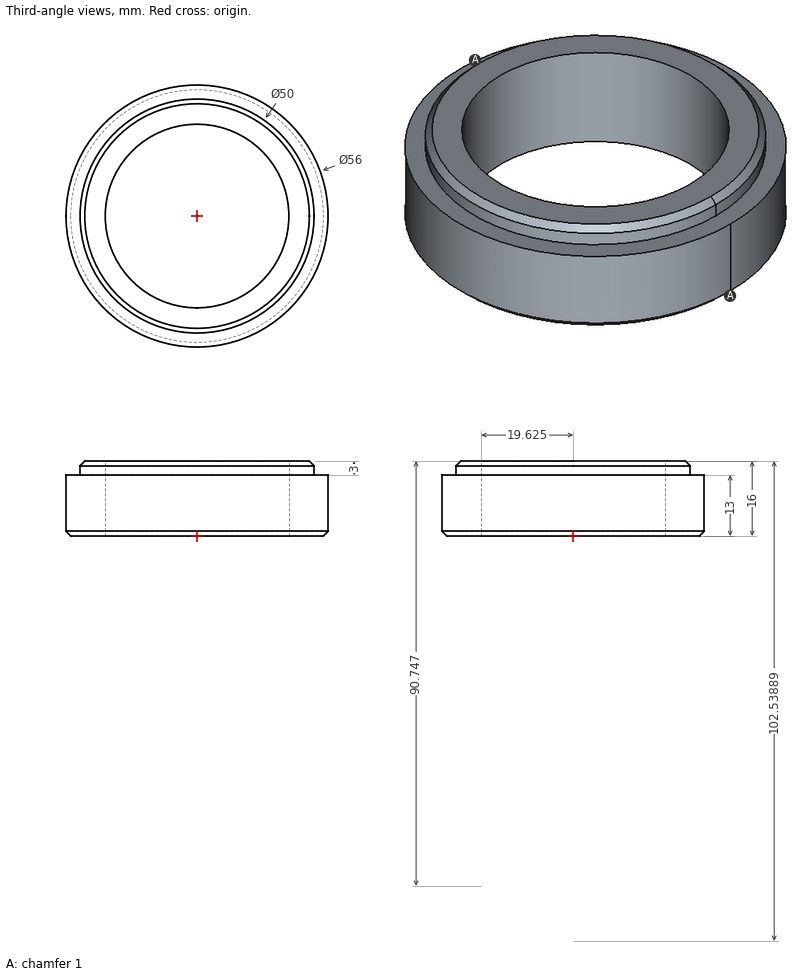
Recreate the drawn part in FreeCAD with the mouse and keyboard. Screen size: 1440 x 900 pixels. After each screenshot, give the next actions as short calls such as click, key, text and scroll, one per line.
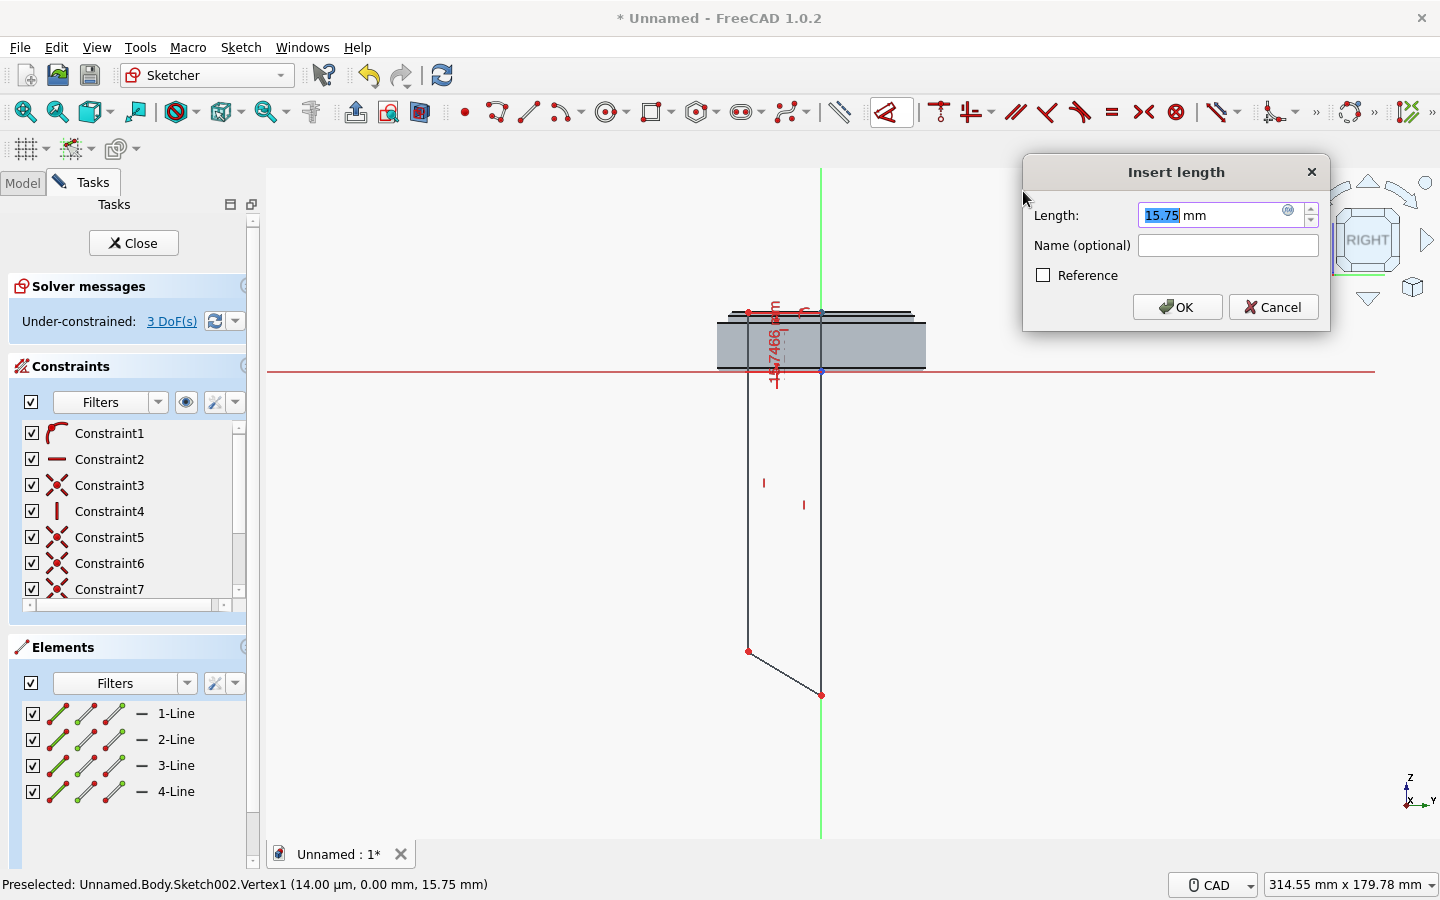
text(16)
key(Return)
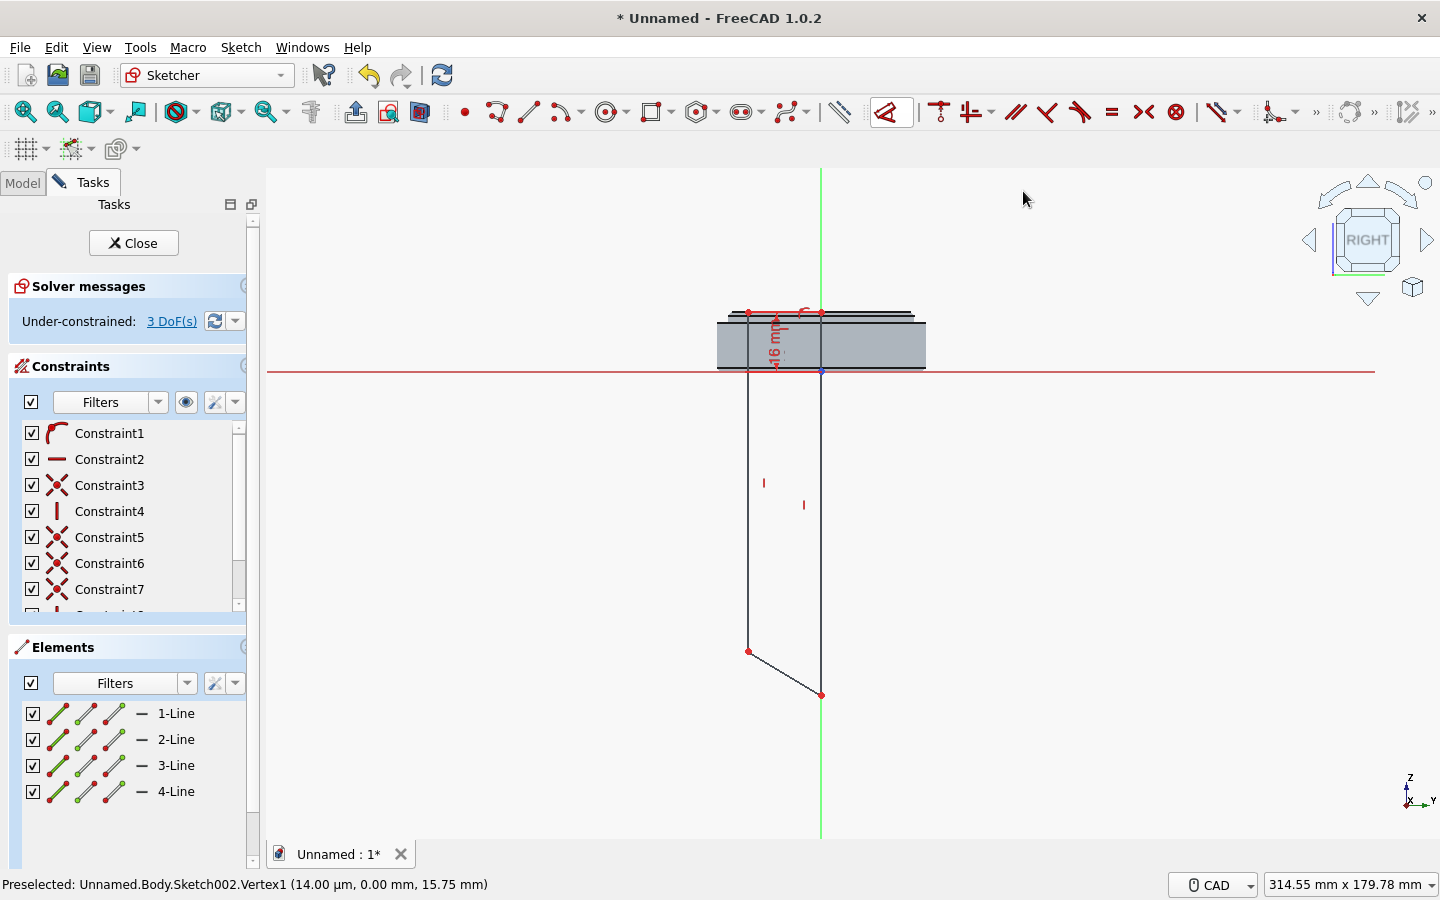
click(770, 312)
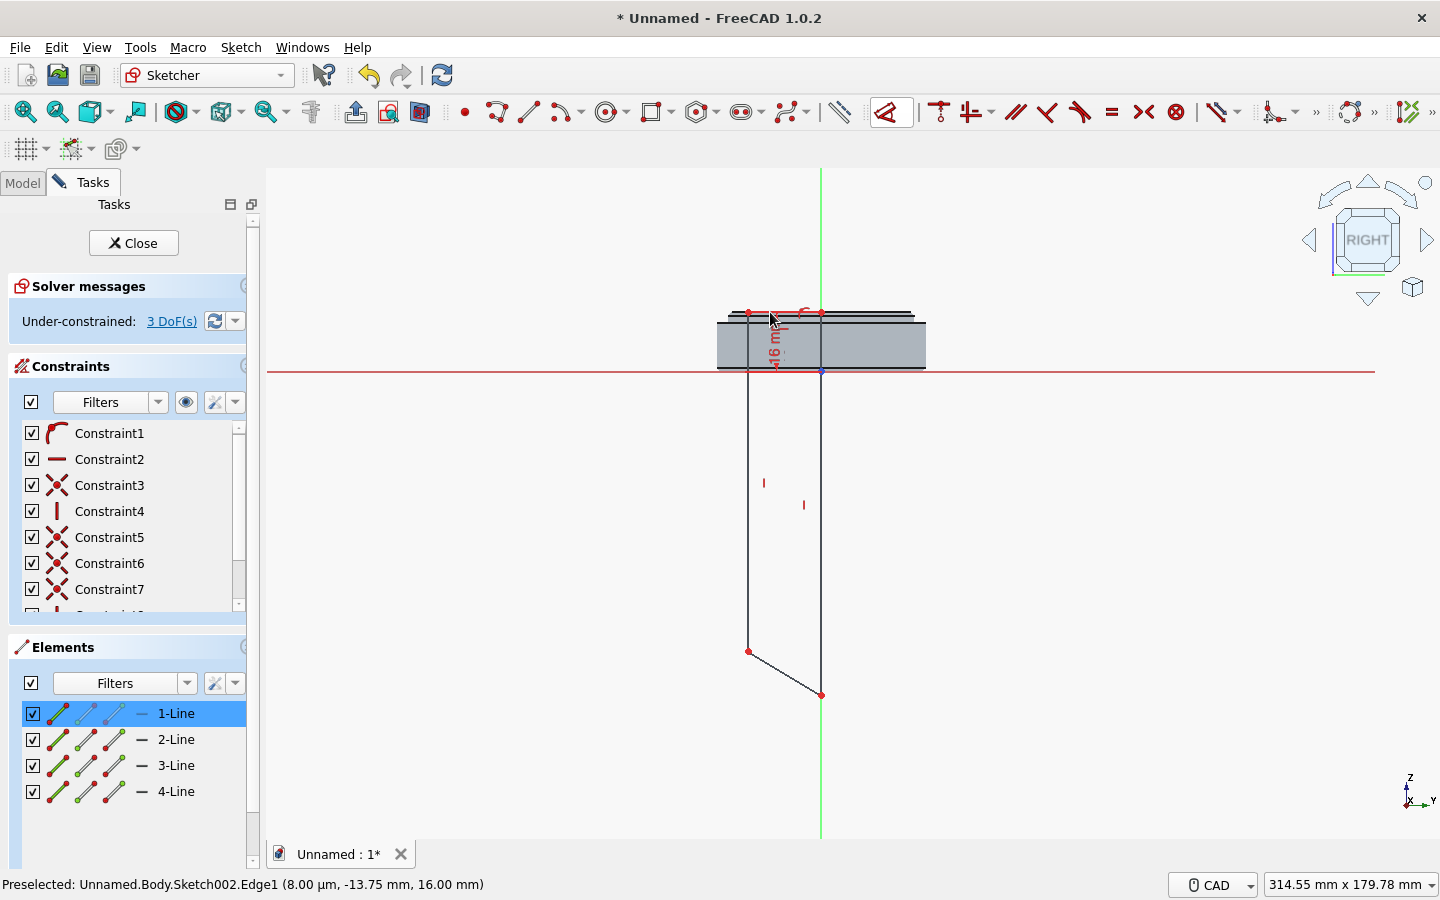
key(l)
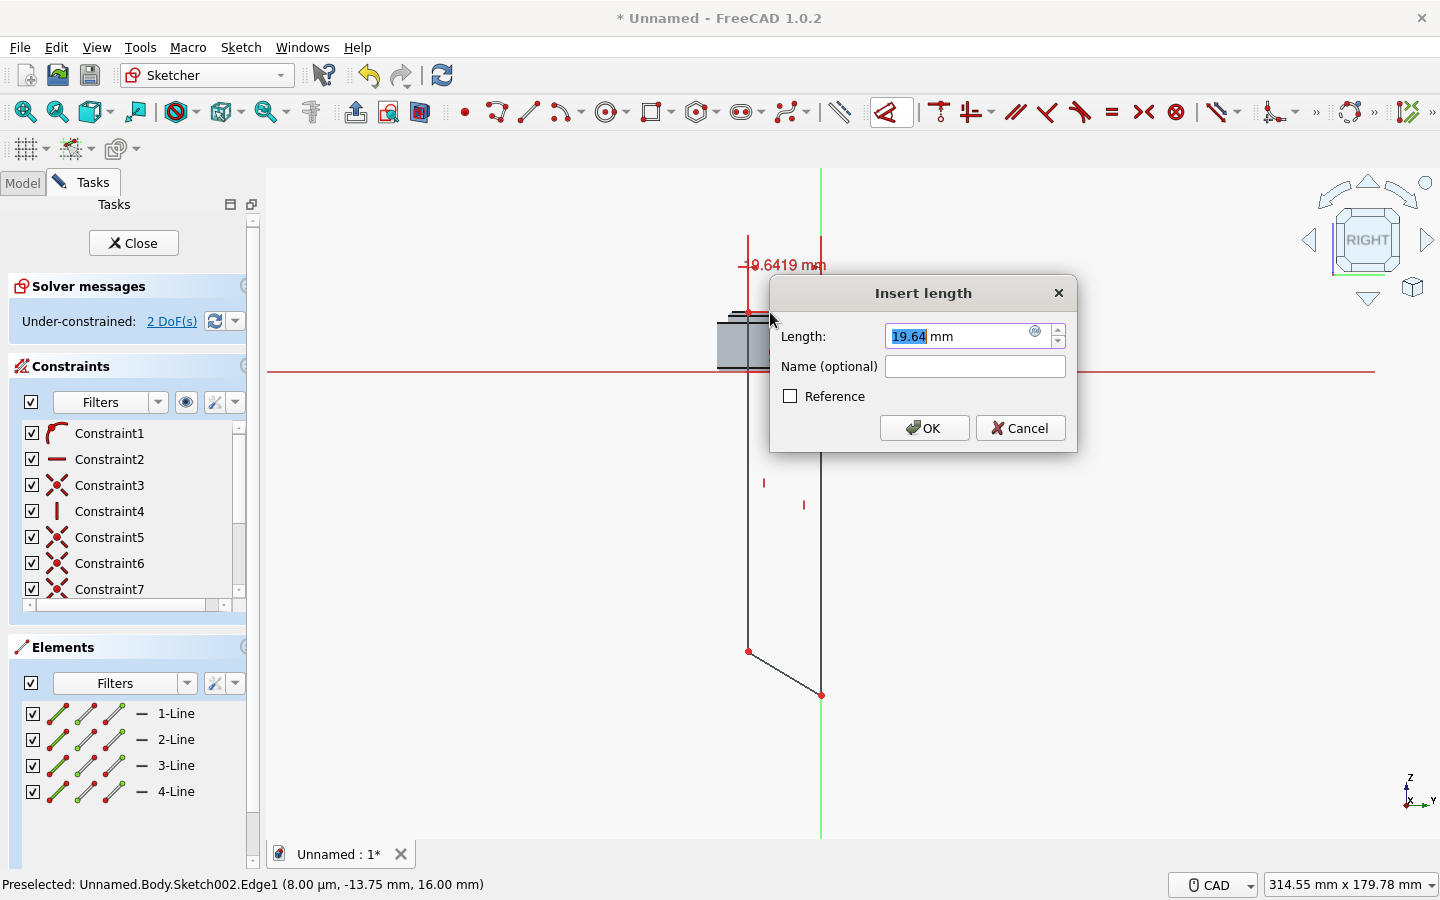
text(19.625)
key(Return)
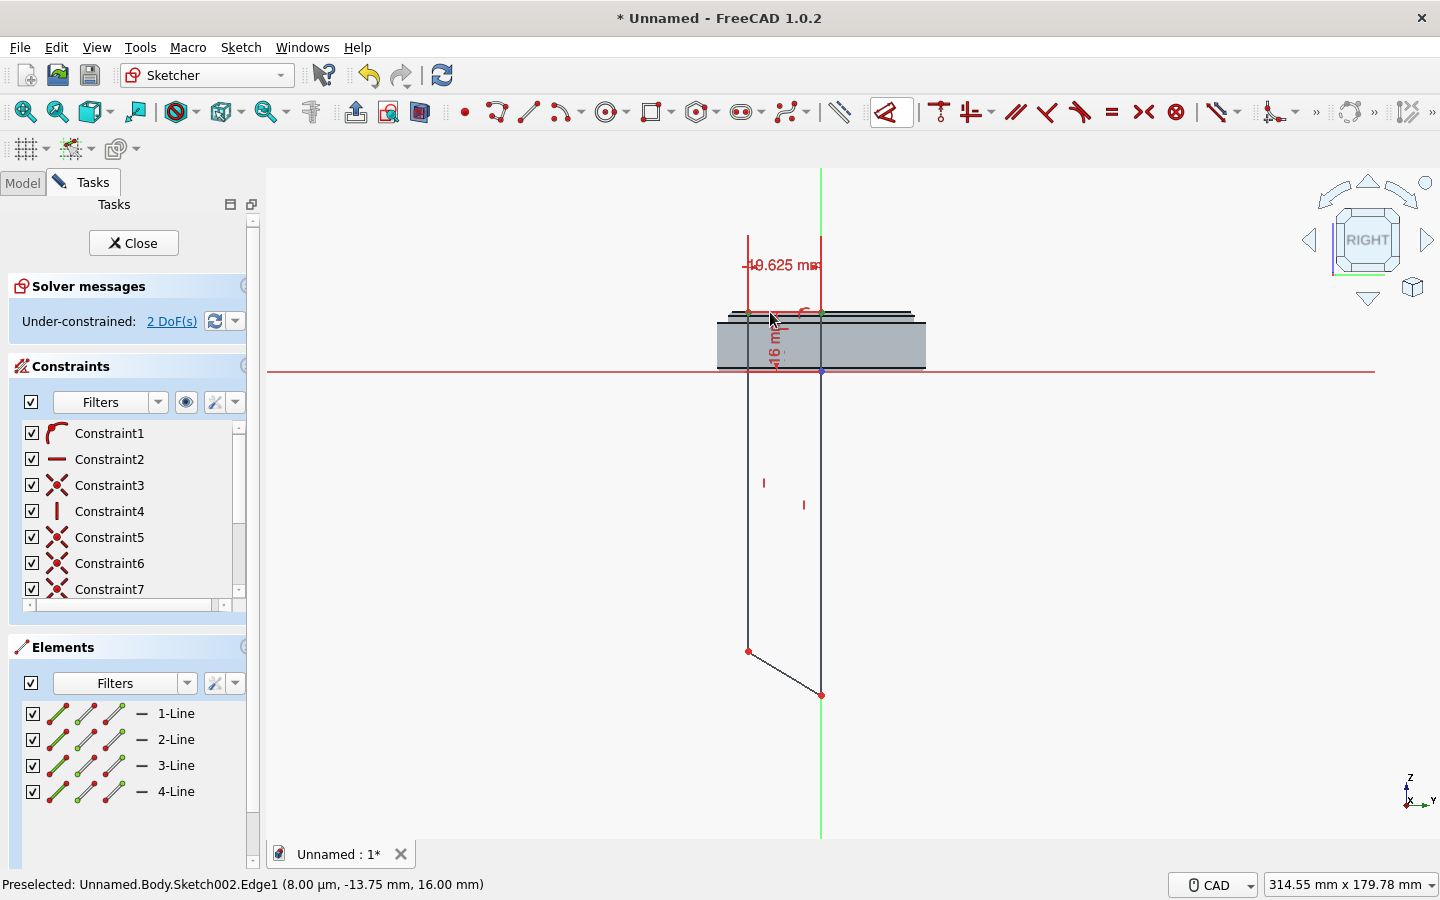
click(748, 414)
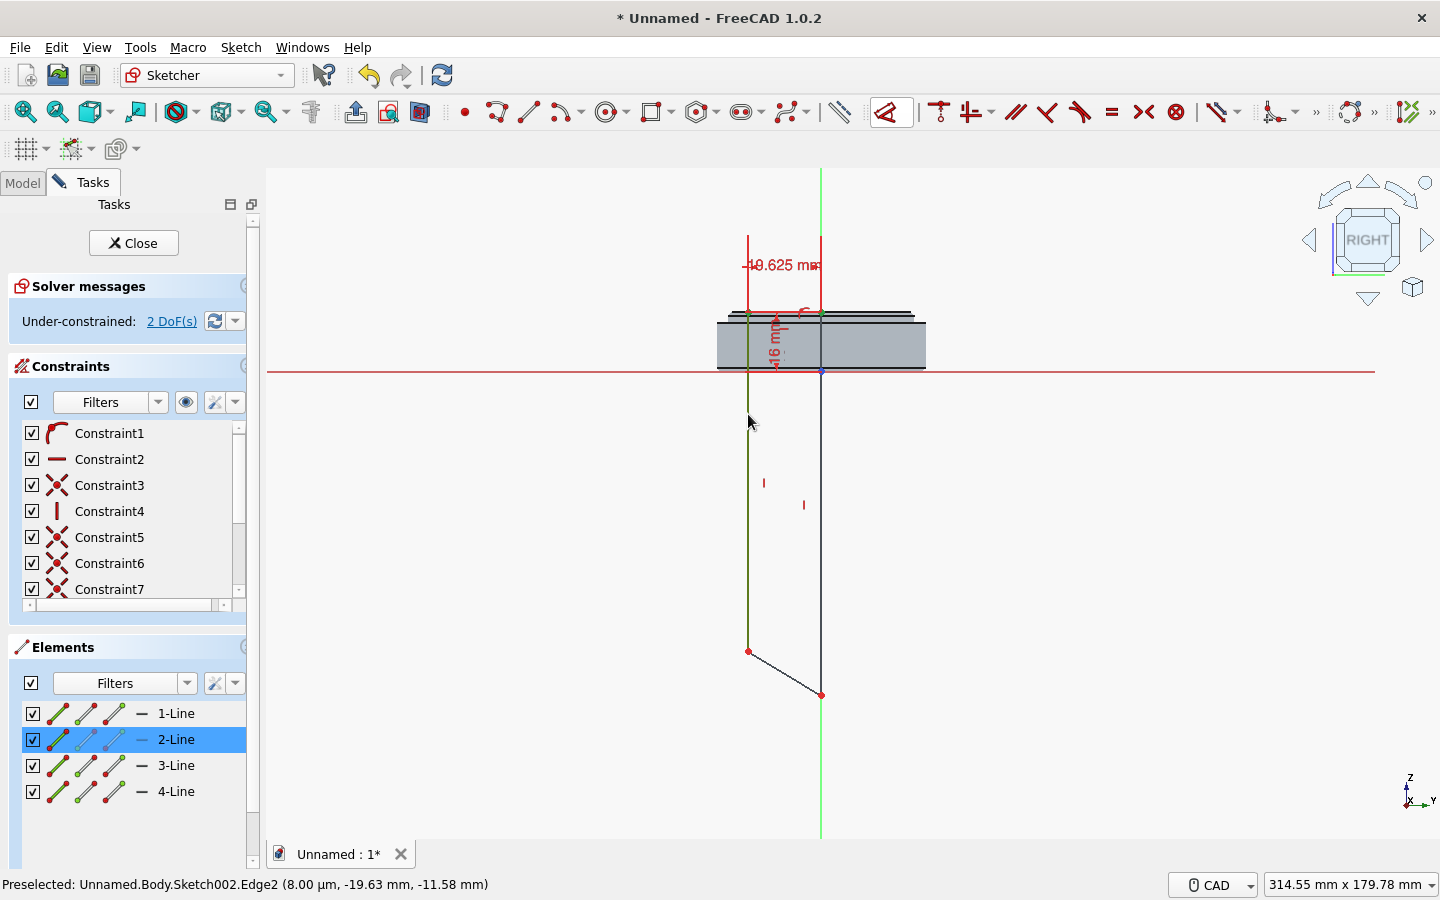
key(i)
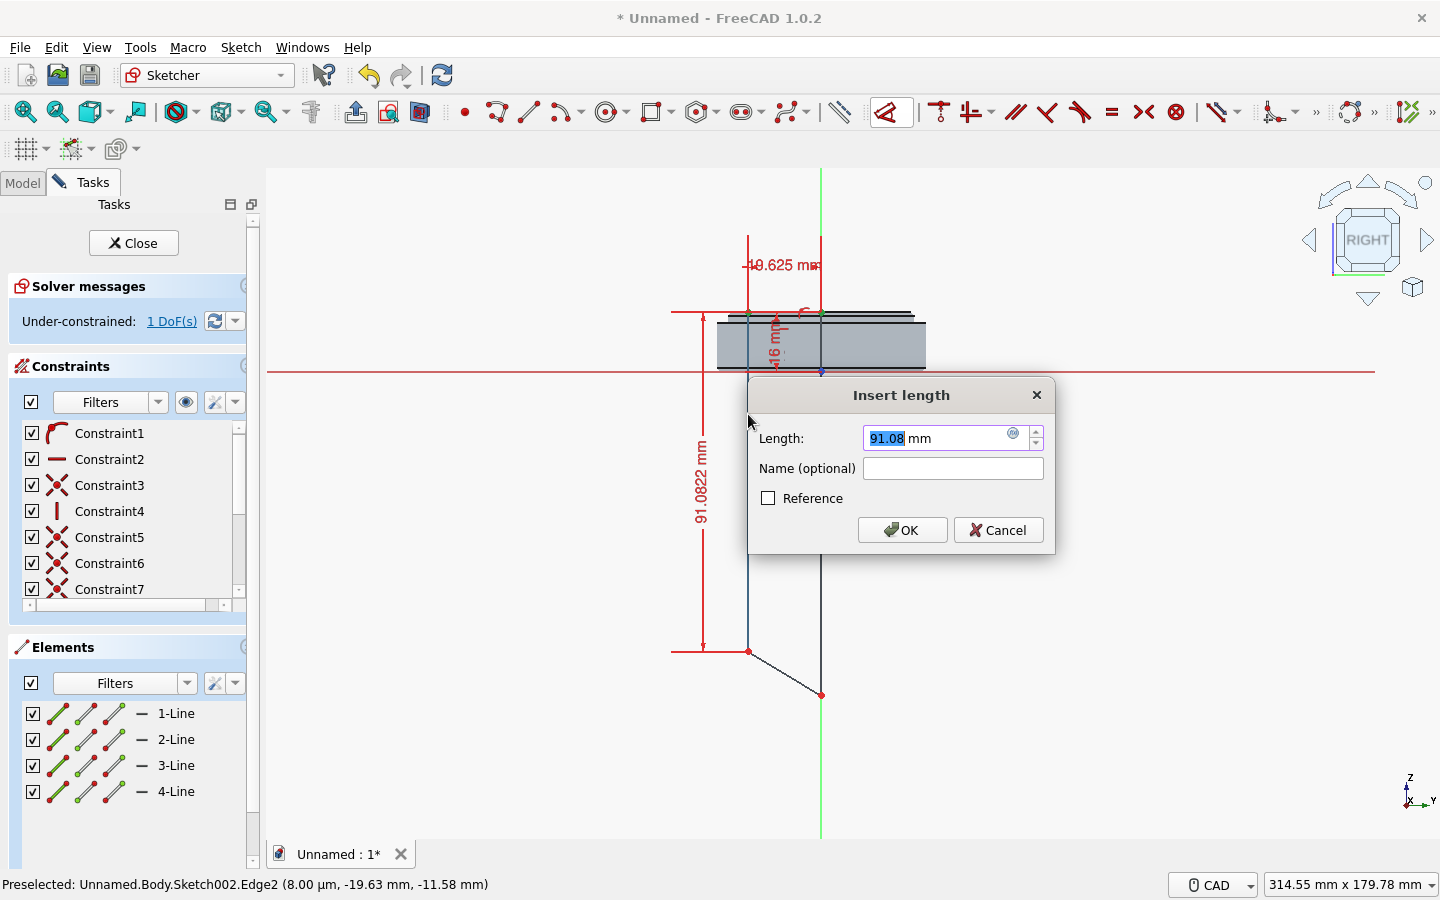
text(90.747)
key(Return)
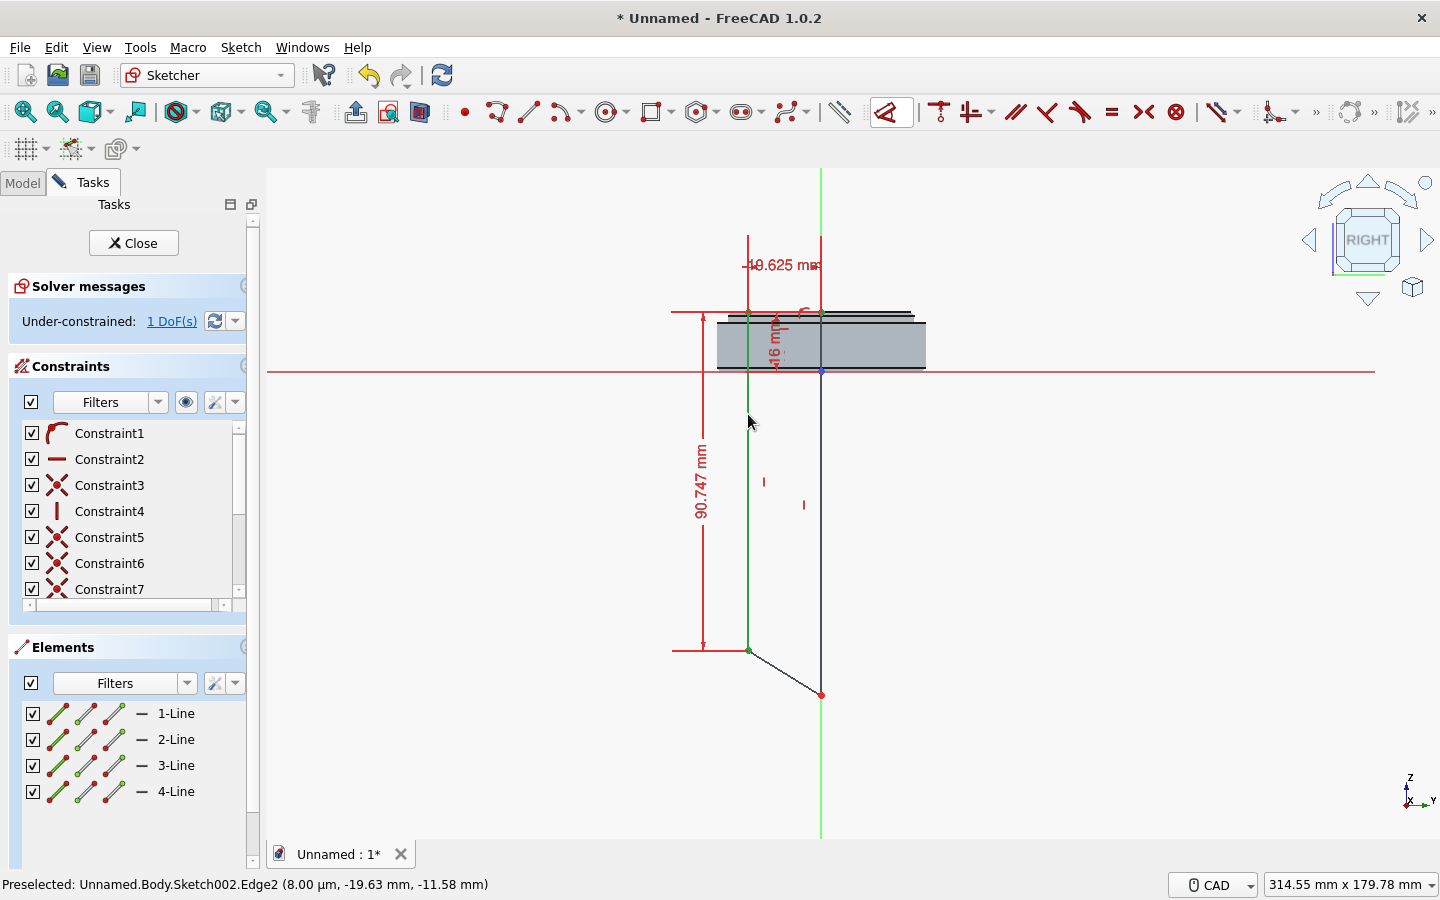
click(821, 581)